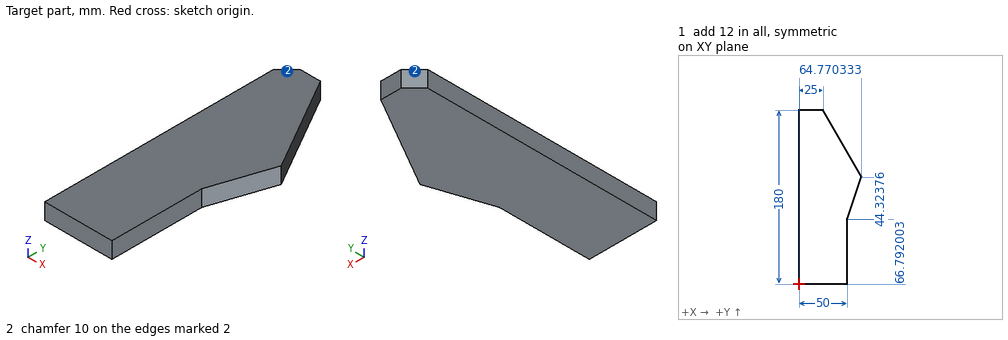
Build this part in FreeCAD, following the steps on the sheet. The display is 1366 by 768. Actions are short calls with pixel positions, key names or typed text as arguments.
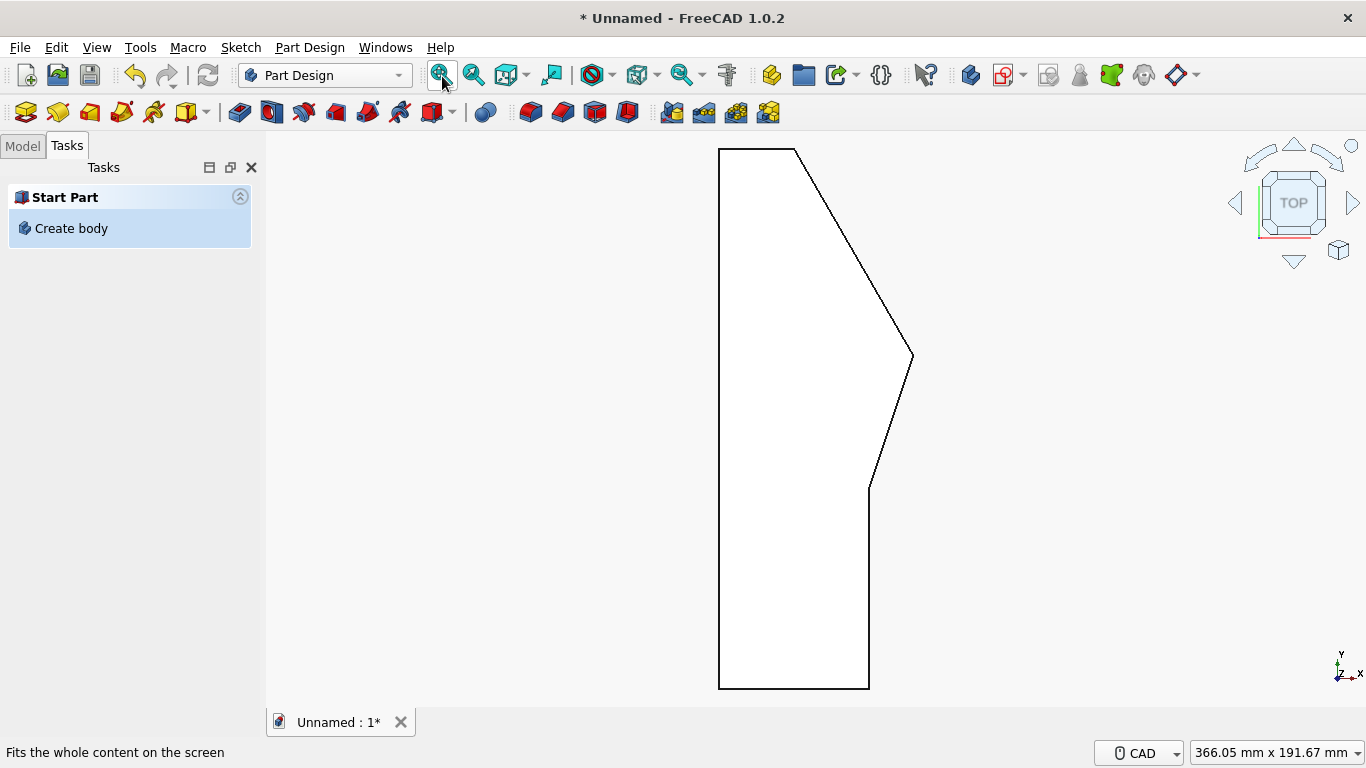
key(1)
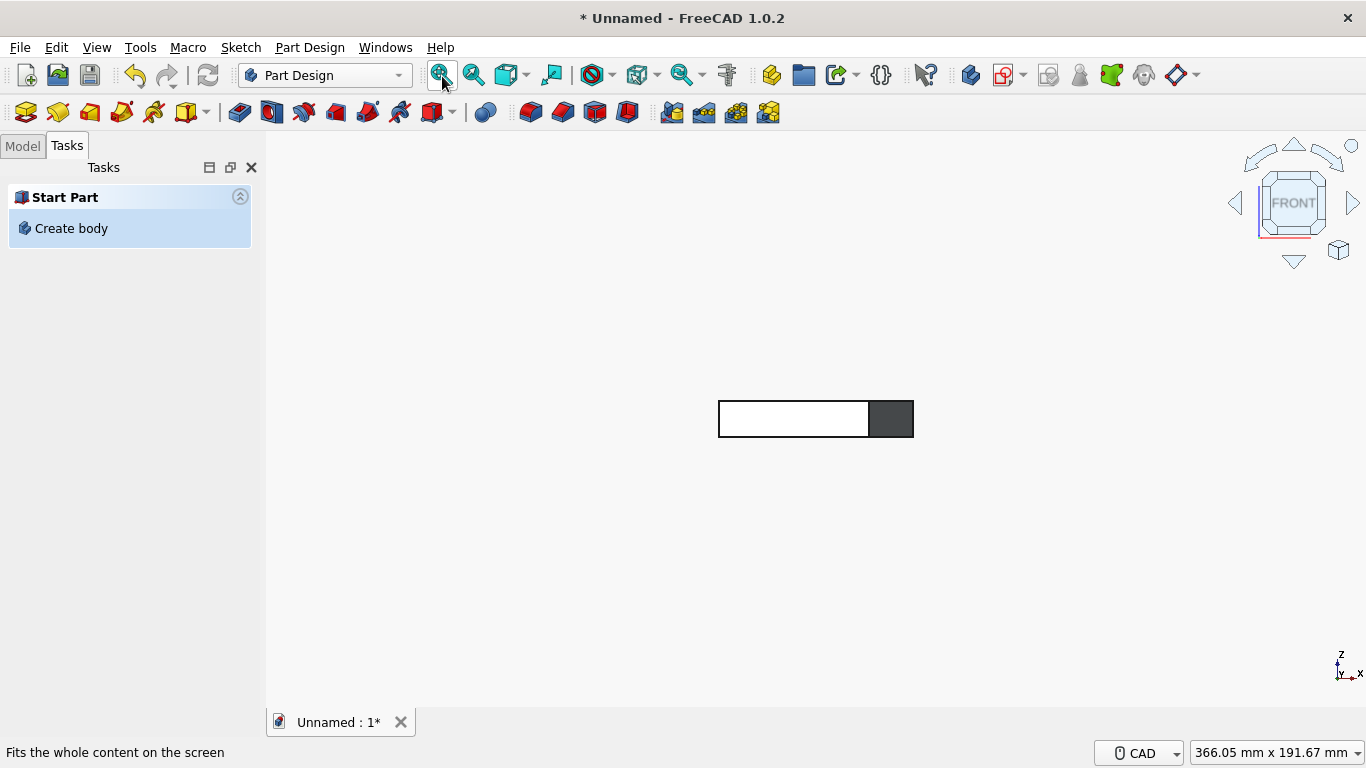
click(442, 76)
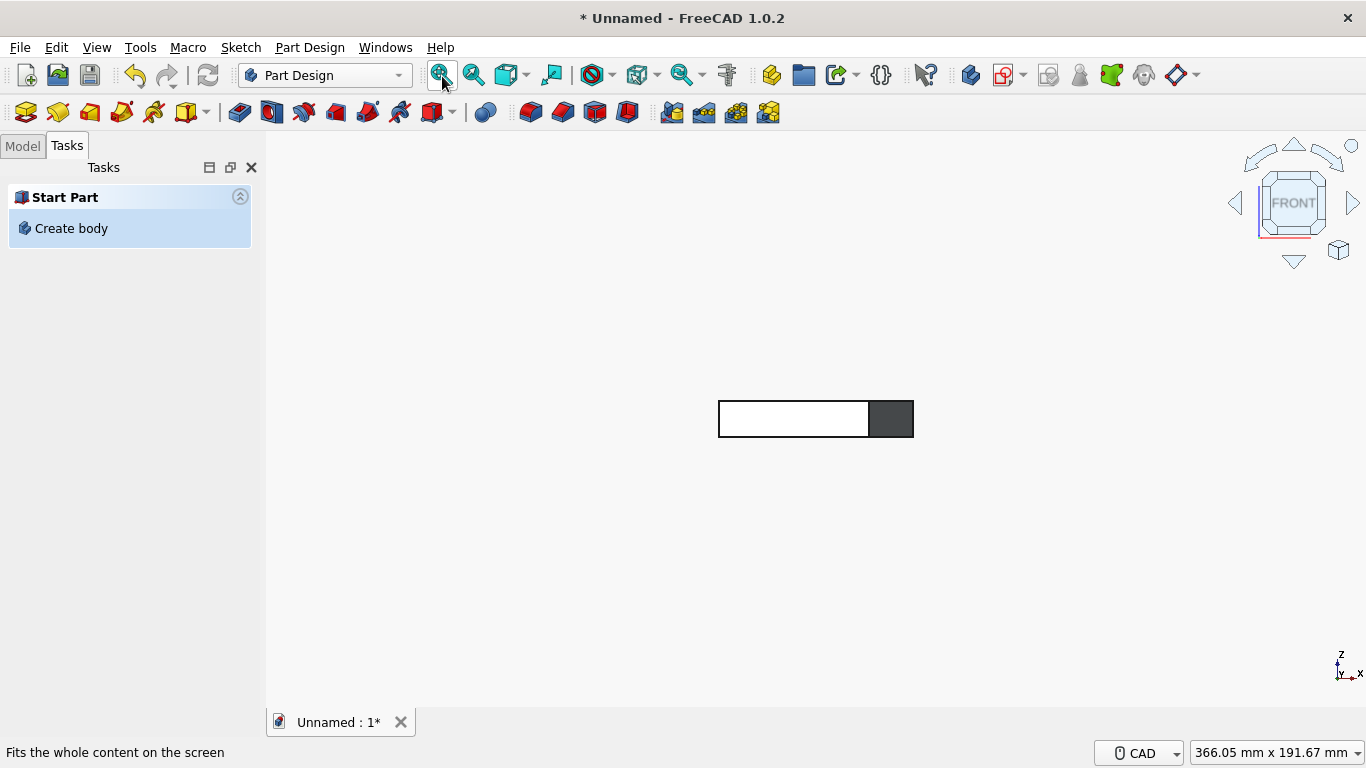
key(3)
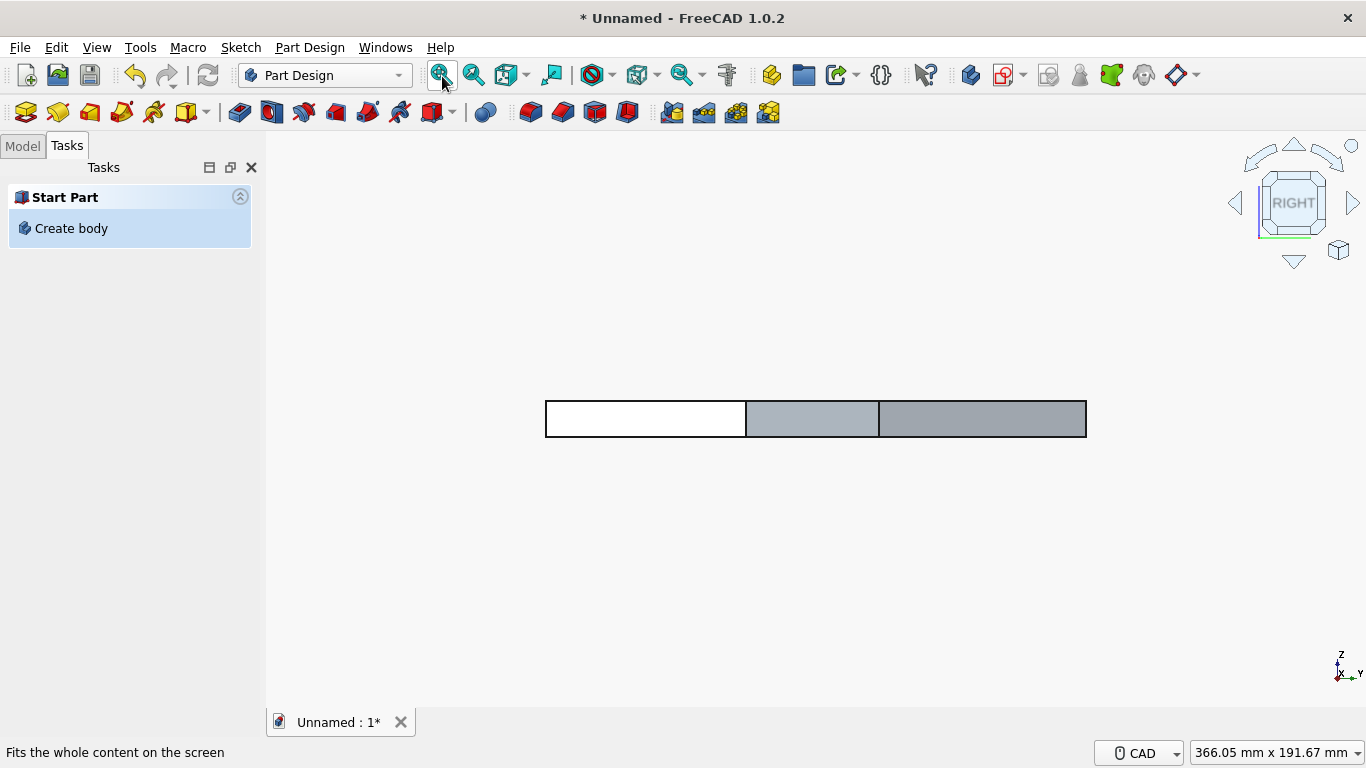
key(5)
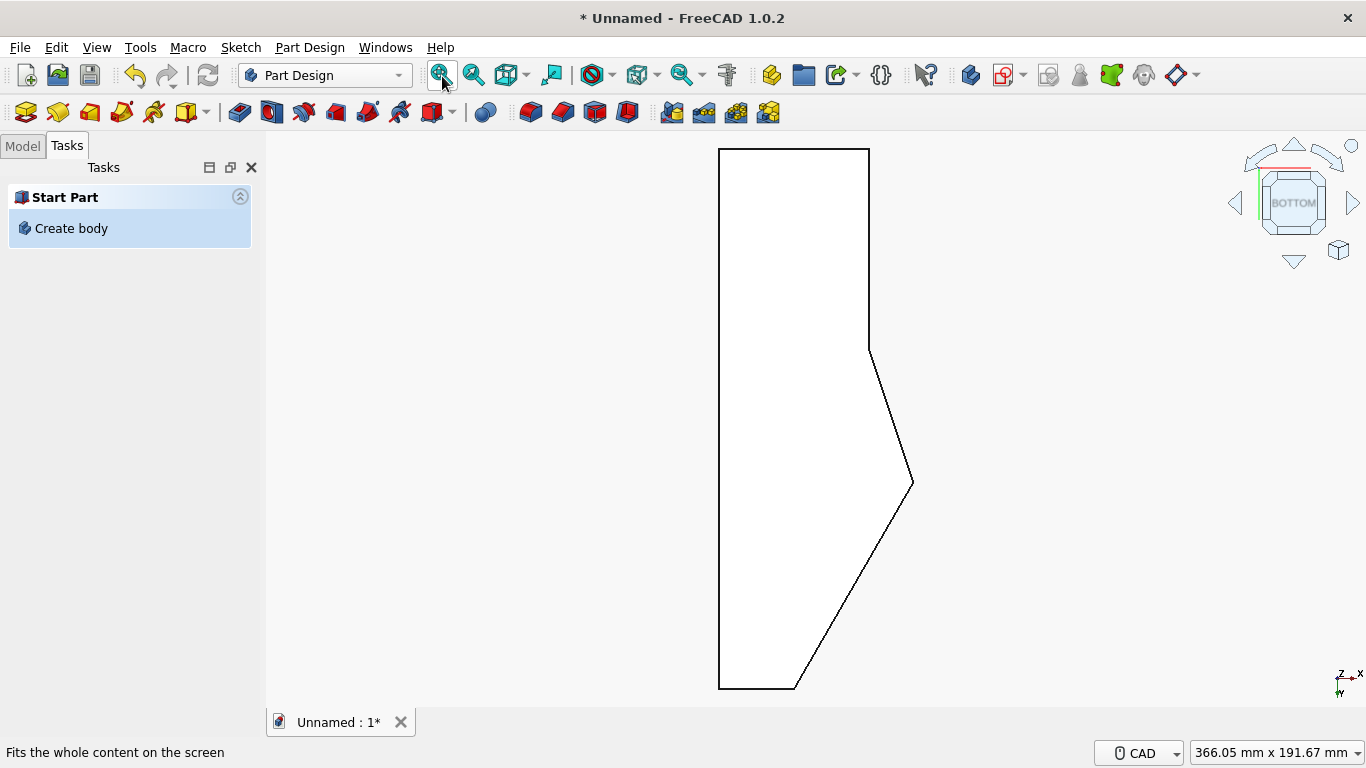
key(4)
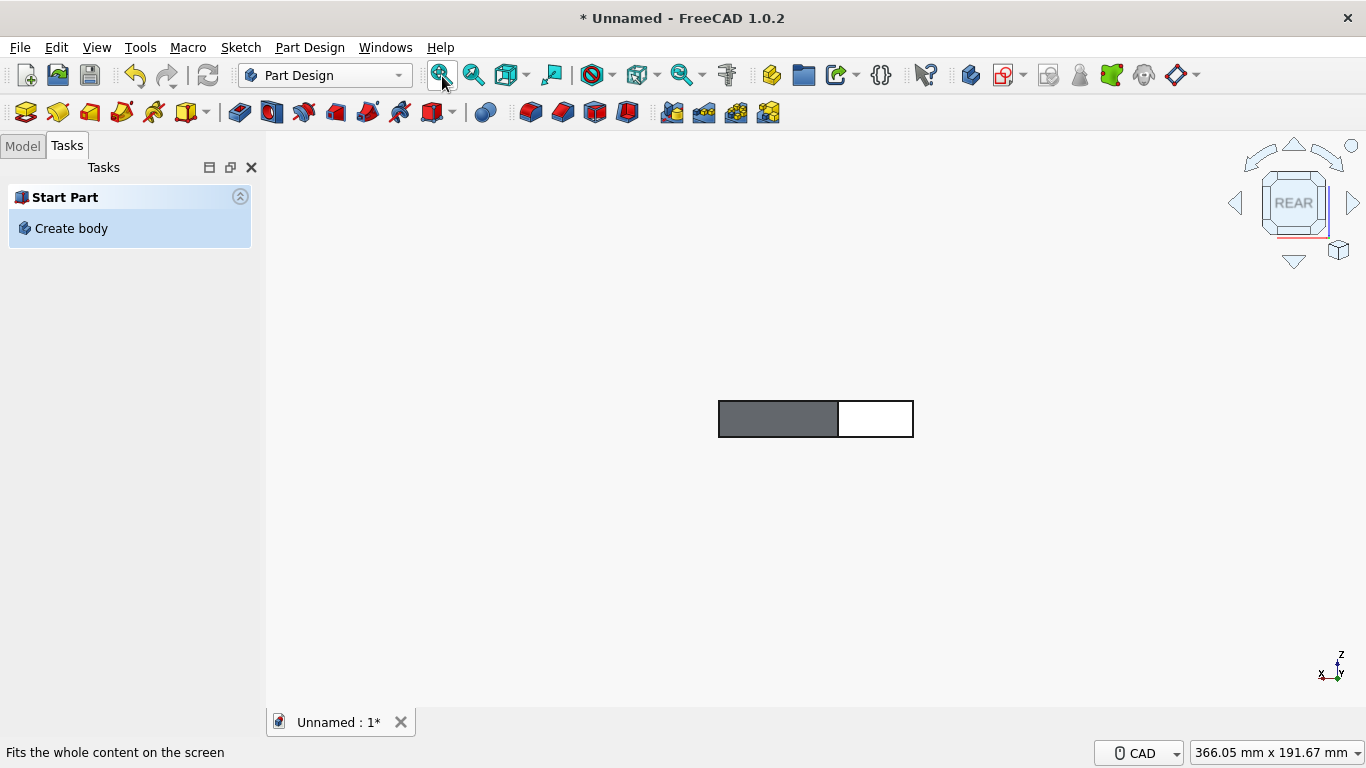
key(v)
key(f)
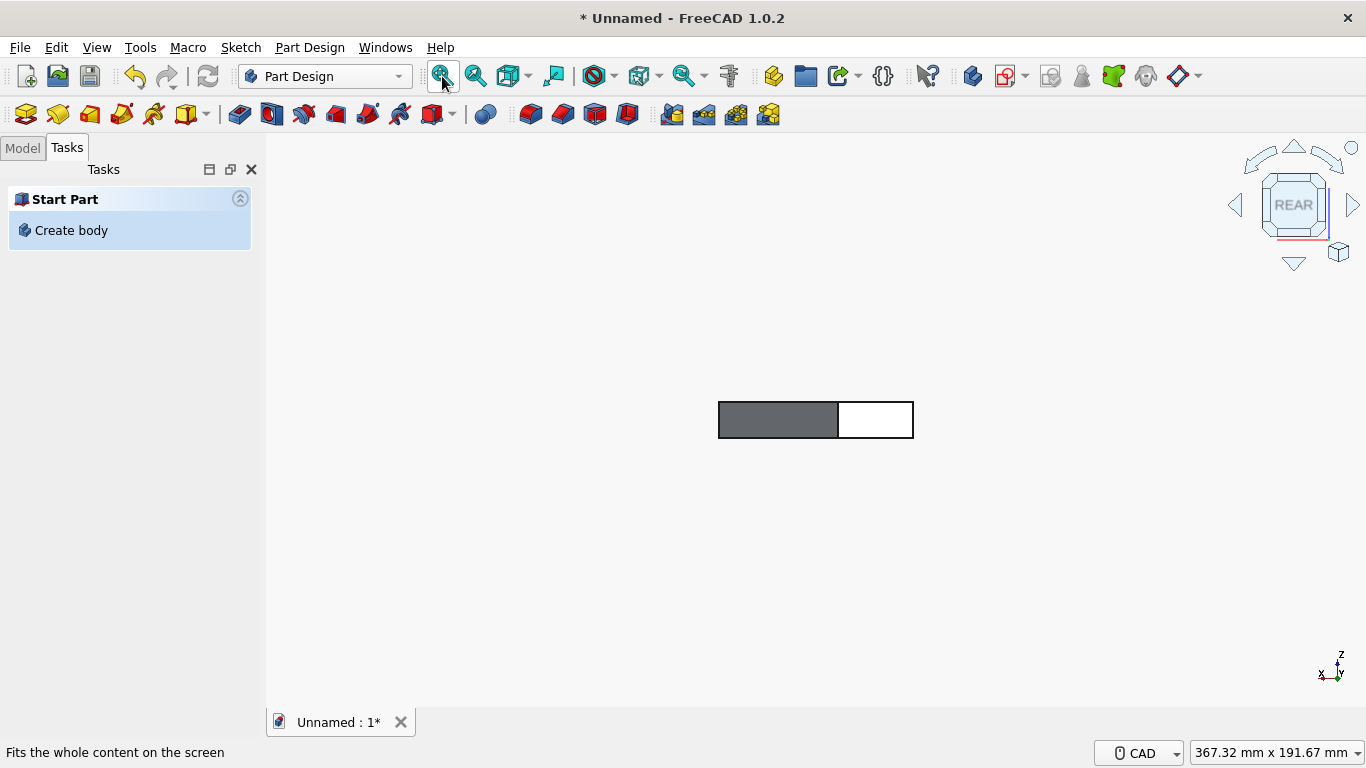
click(913, 419)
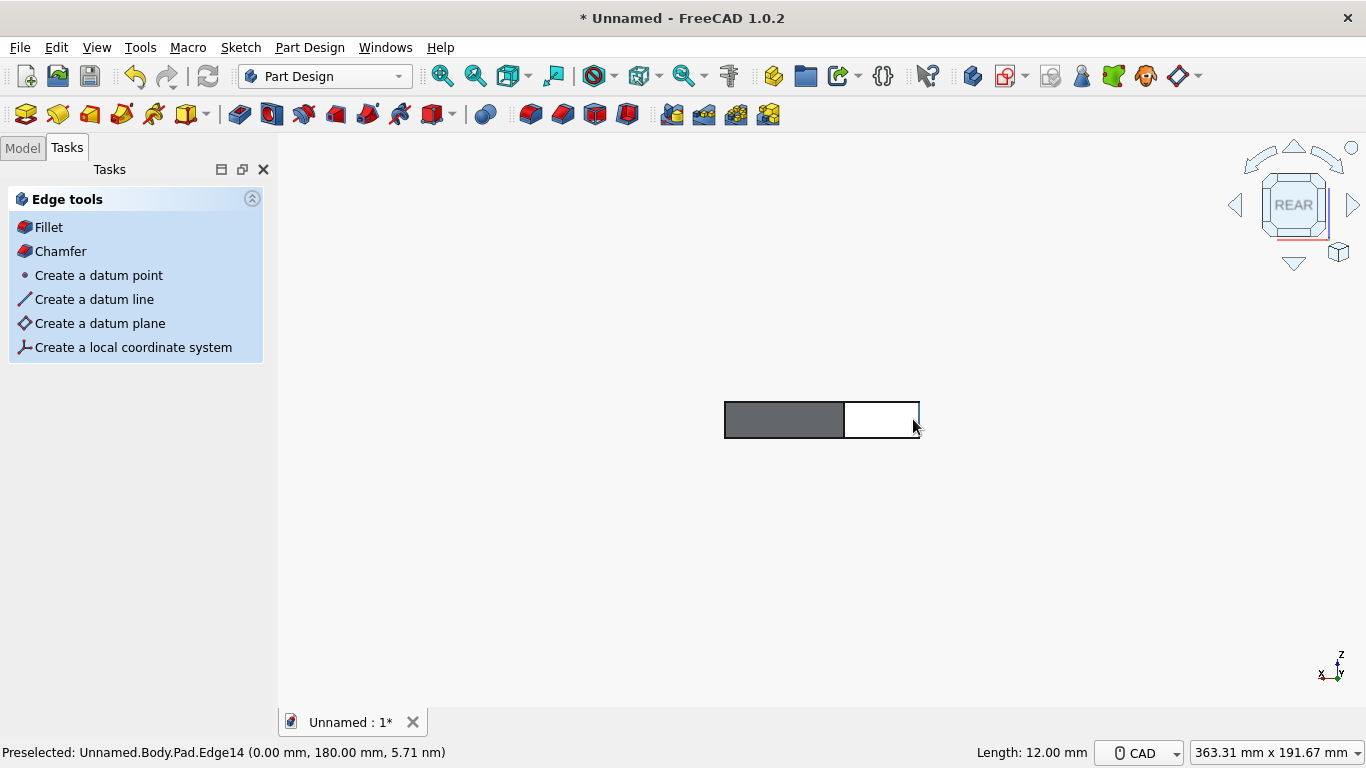
click(564, 114)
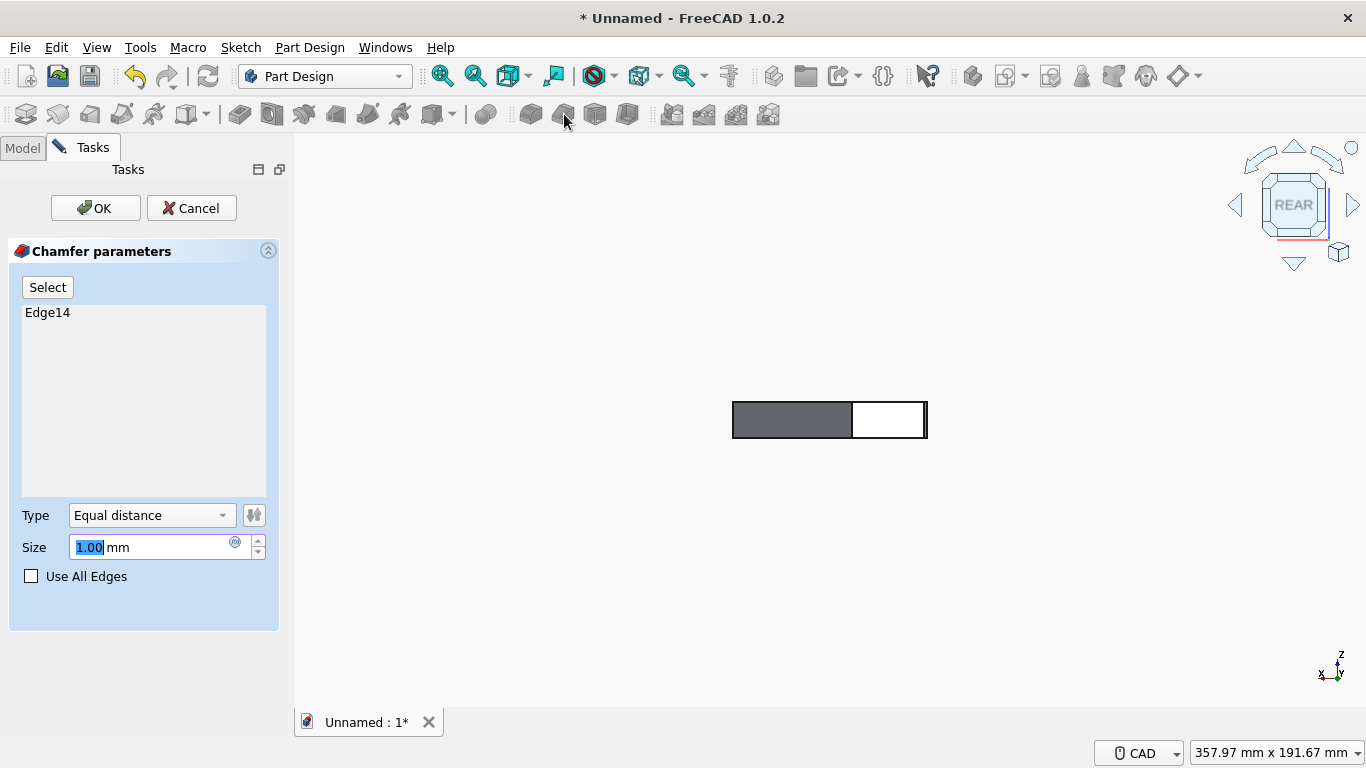
text(10)
key(Tab)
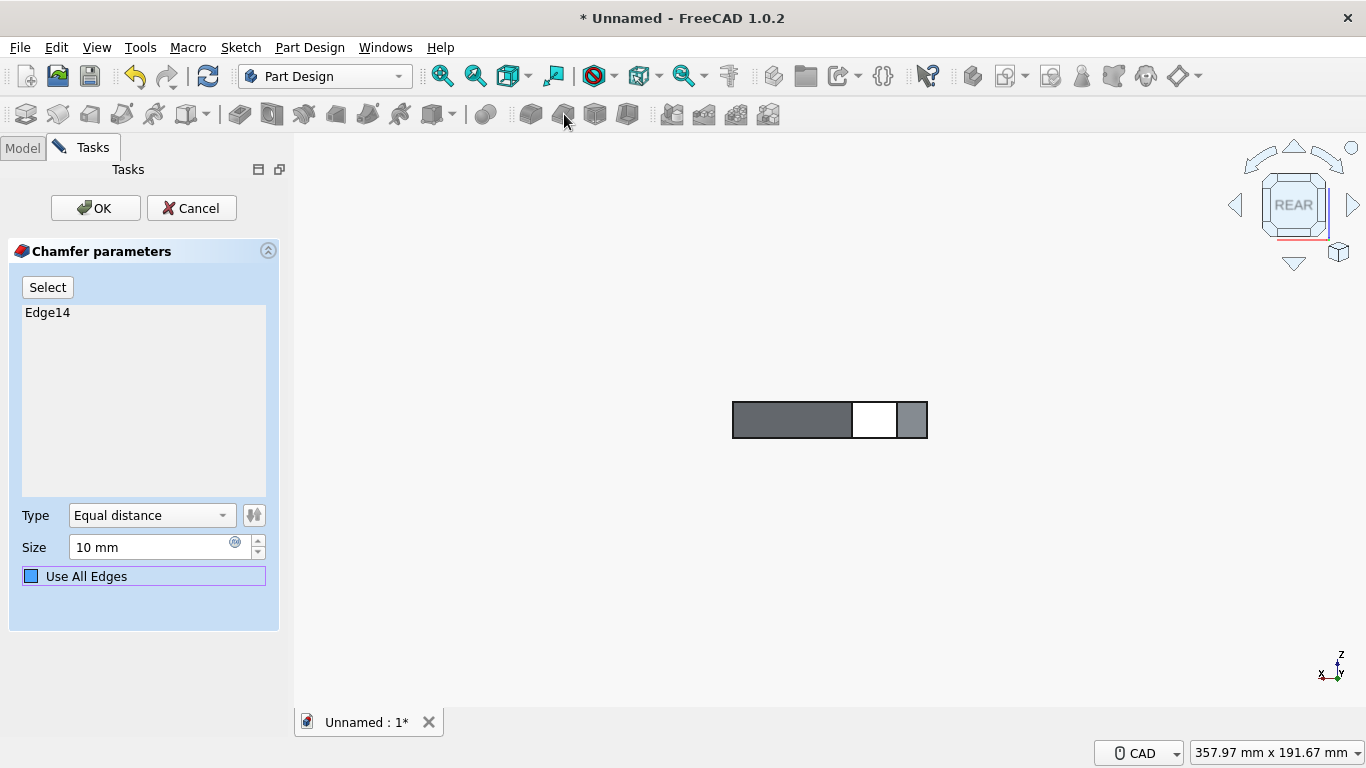
click(96, 208)